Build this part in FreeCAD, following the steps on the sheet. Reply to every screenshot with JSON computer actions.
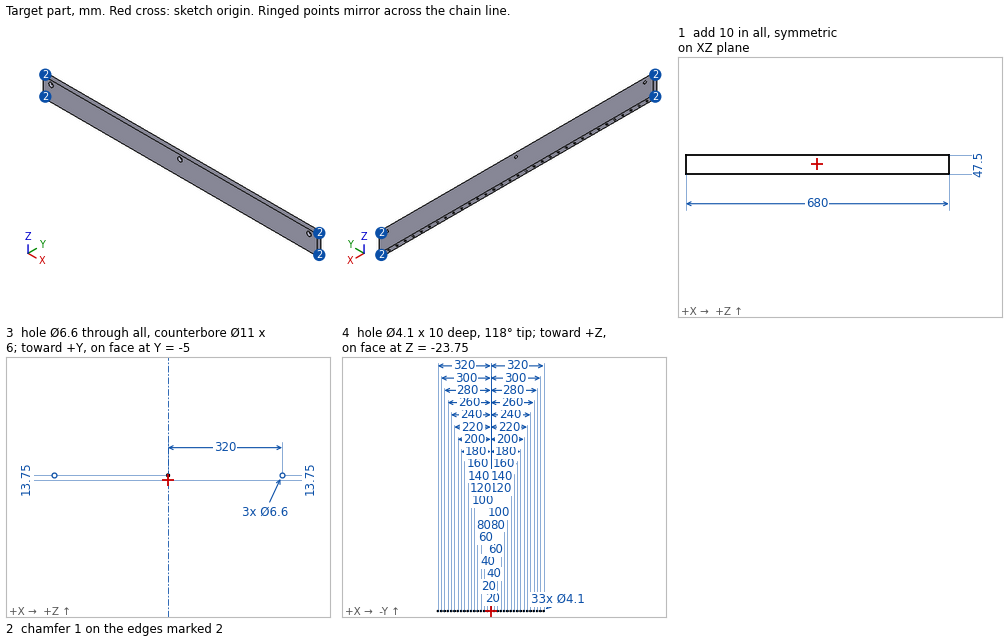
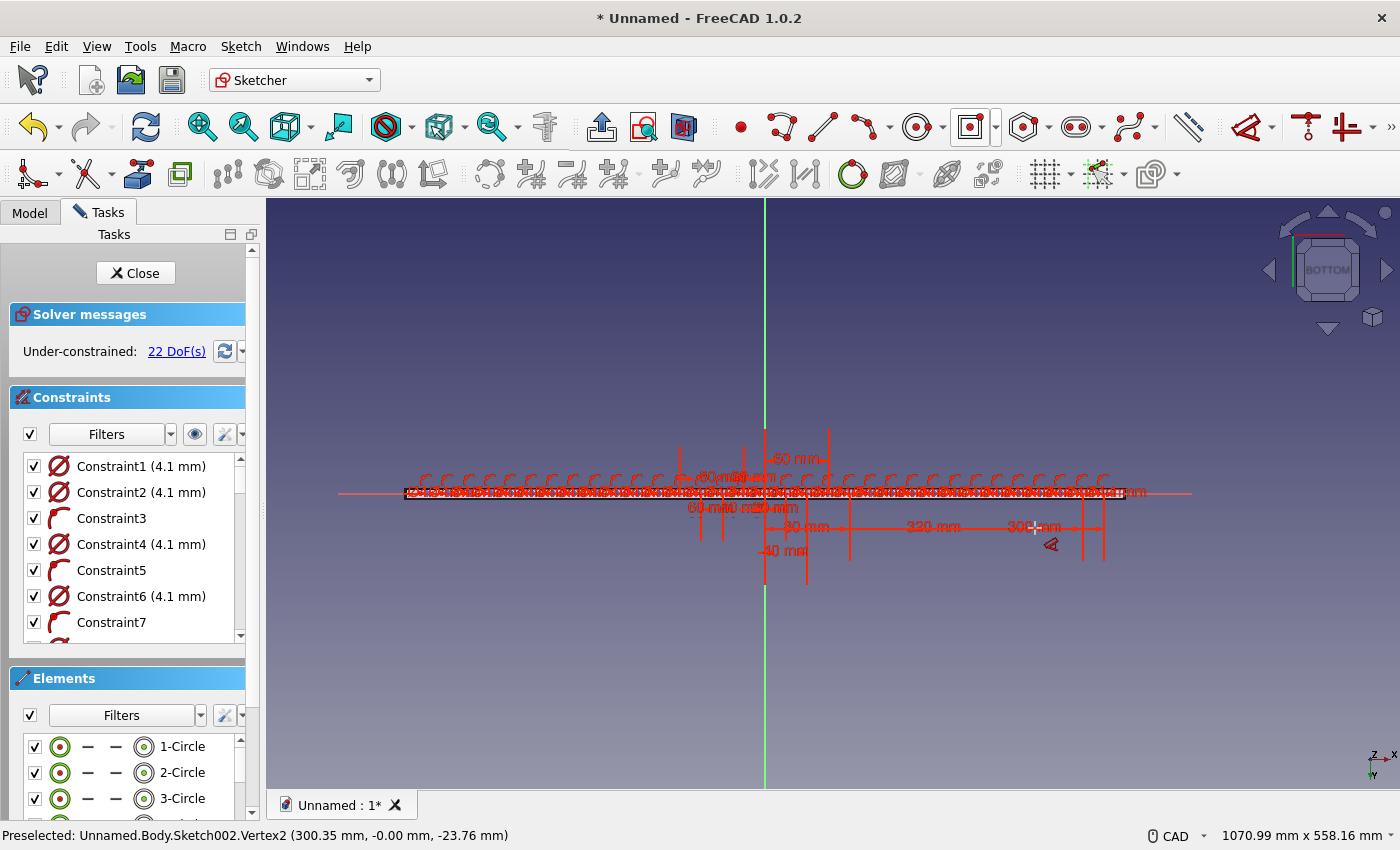
{"action": "left_click", "coordinate": [1061, 494]}
{"action": "left_click", "coordinate": [913, 460]}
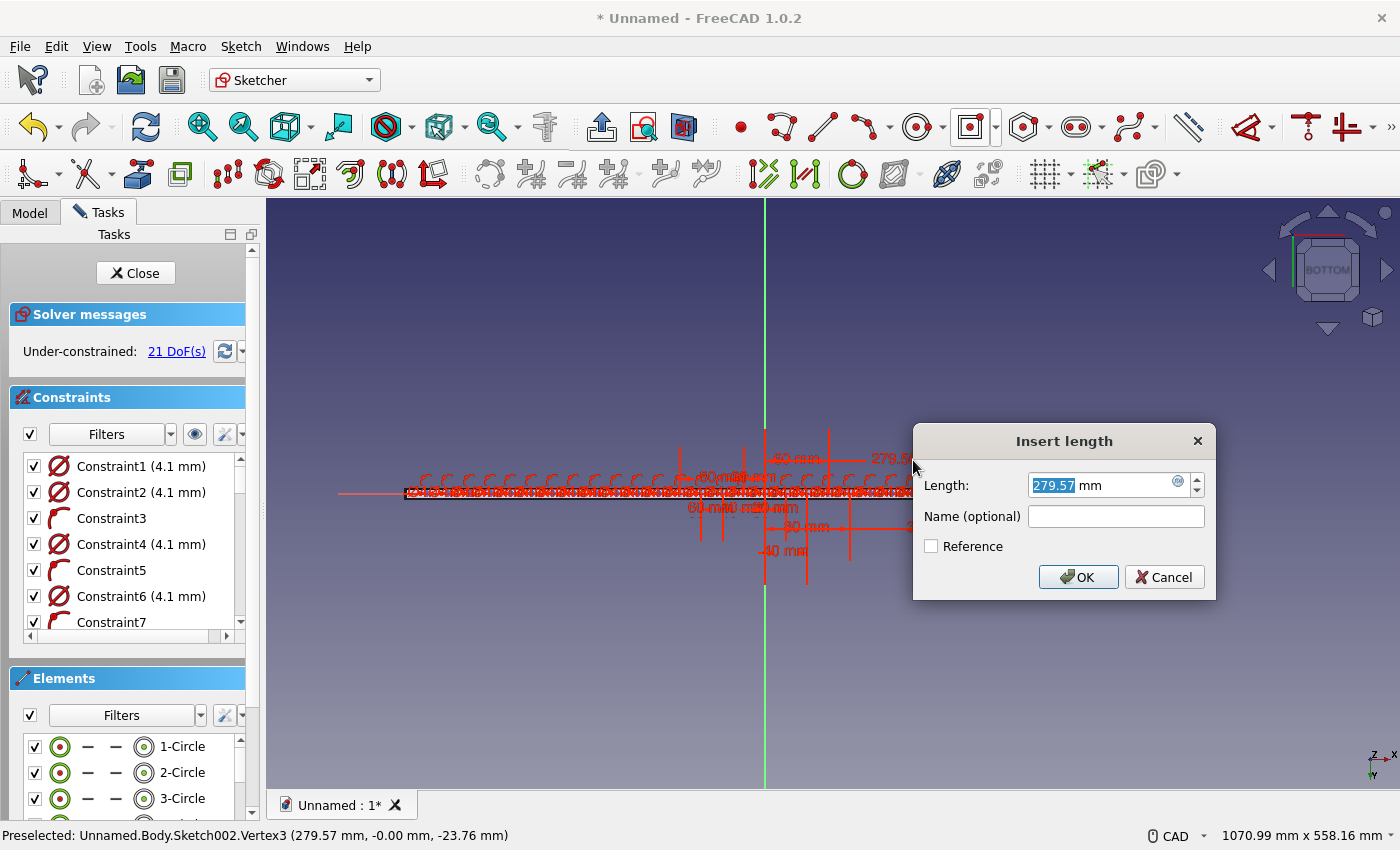
{"action": "type", "text": "280"}
{"action": "key", "text": "Return"}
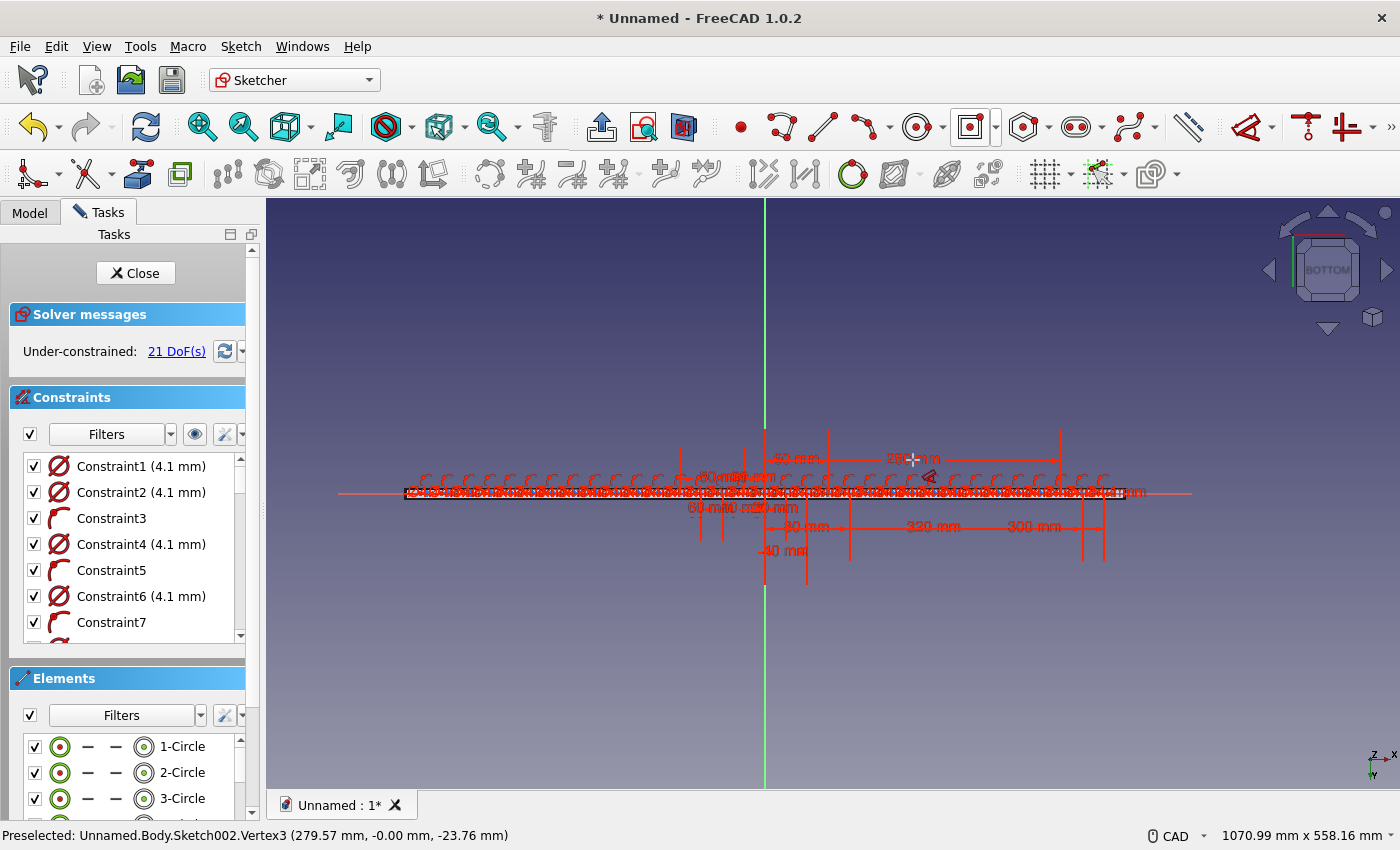
{"action": "left_click", "coordinate": [1040, 494]}
{"action": "left_click", "coordinate": [999, 460]}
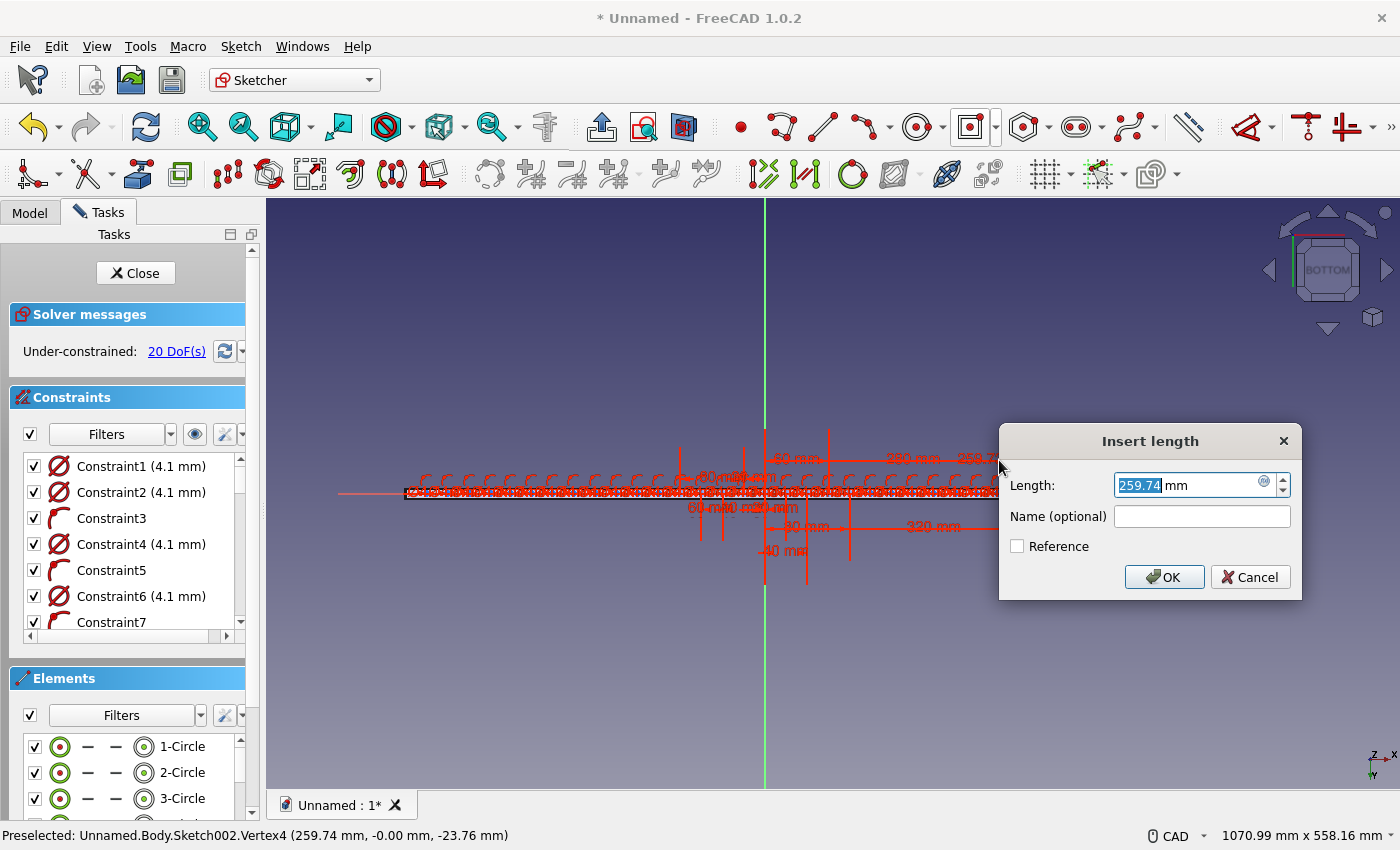
{"action": "type", "text": "260"}
{"action": "key", "text": "Return"}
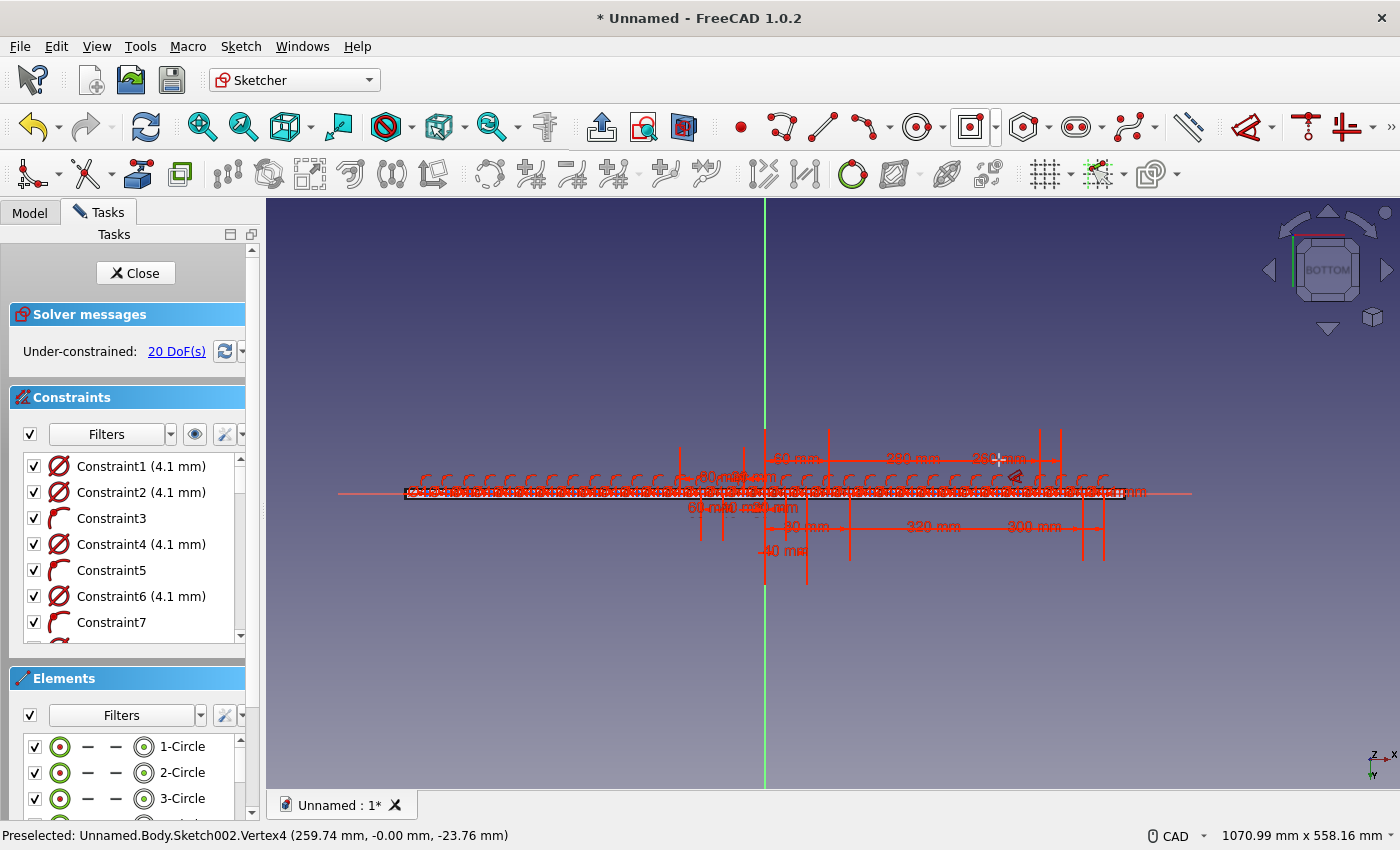
{"action": "left_click", "coordinate": [1019, 494]}
{"action": "left_click", "coordinate": [892, 552]}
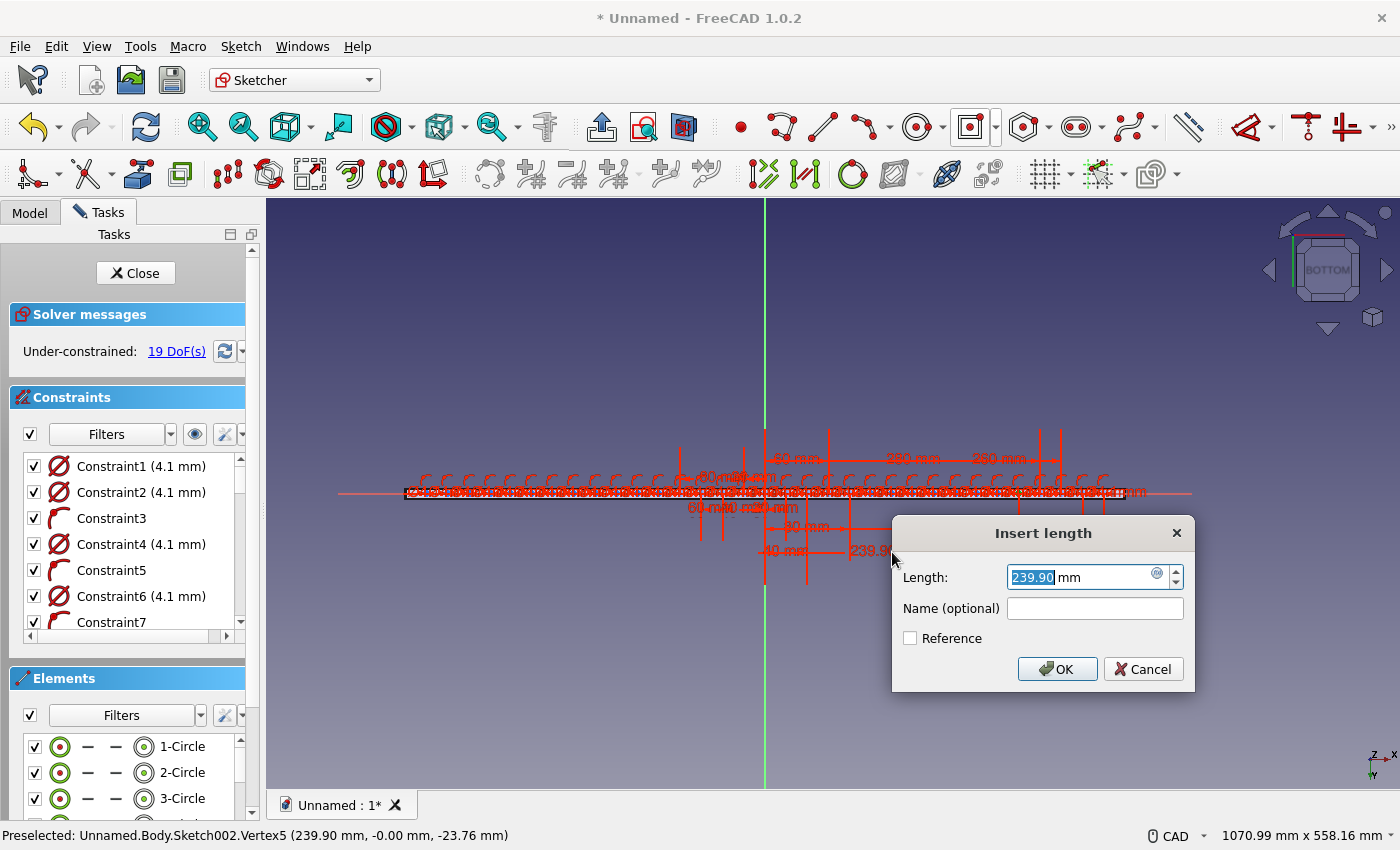
{"action": "type", "text": "240"}
{"action": "key", "text": "Return"}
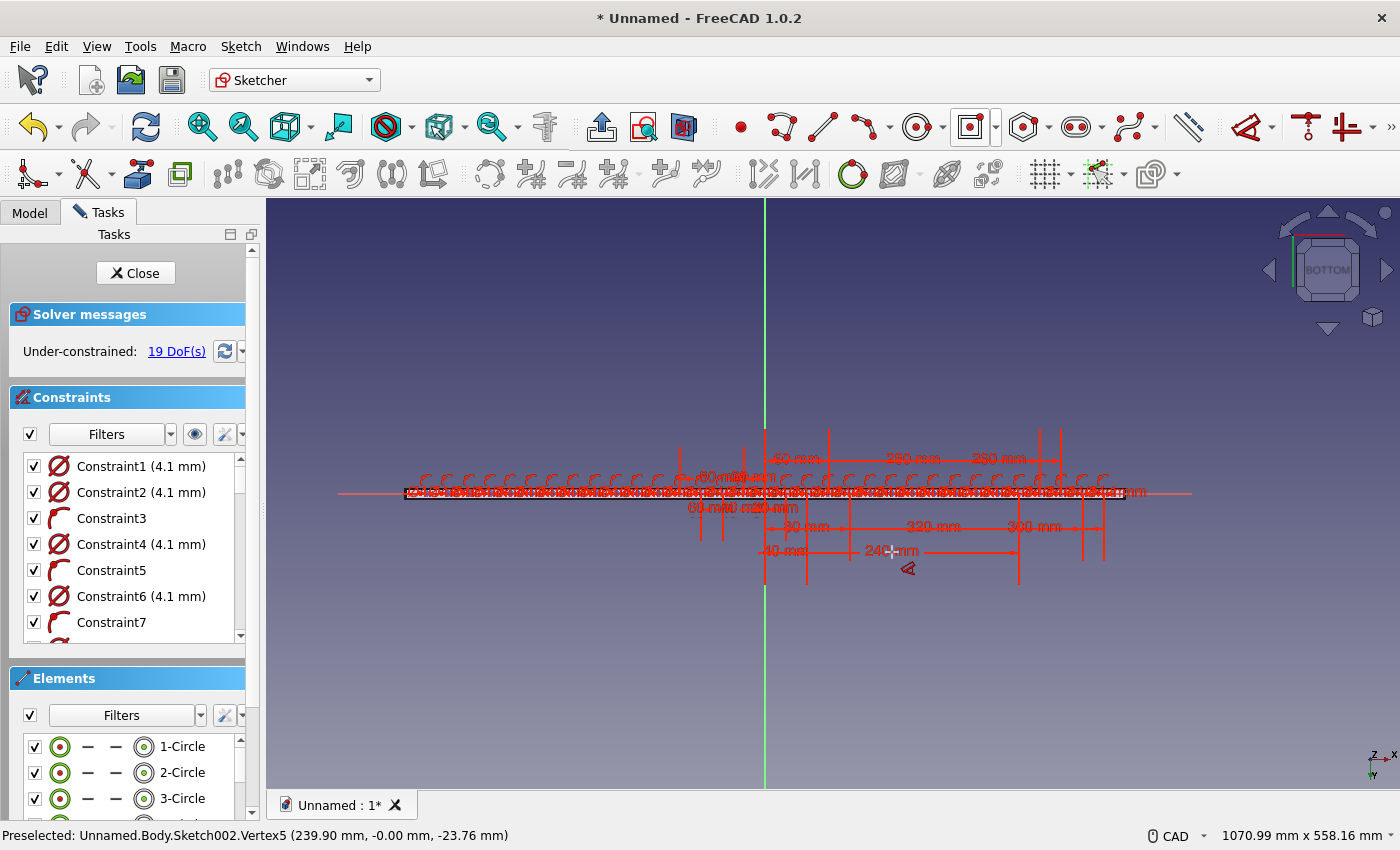
{"action": "left_click", "coordinate": [998, 494]}
{"action": "left_click", "coordinate": [963, 552]}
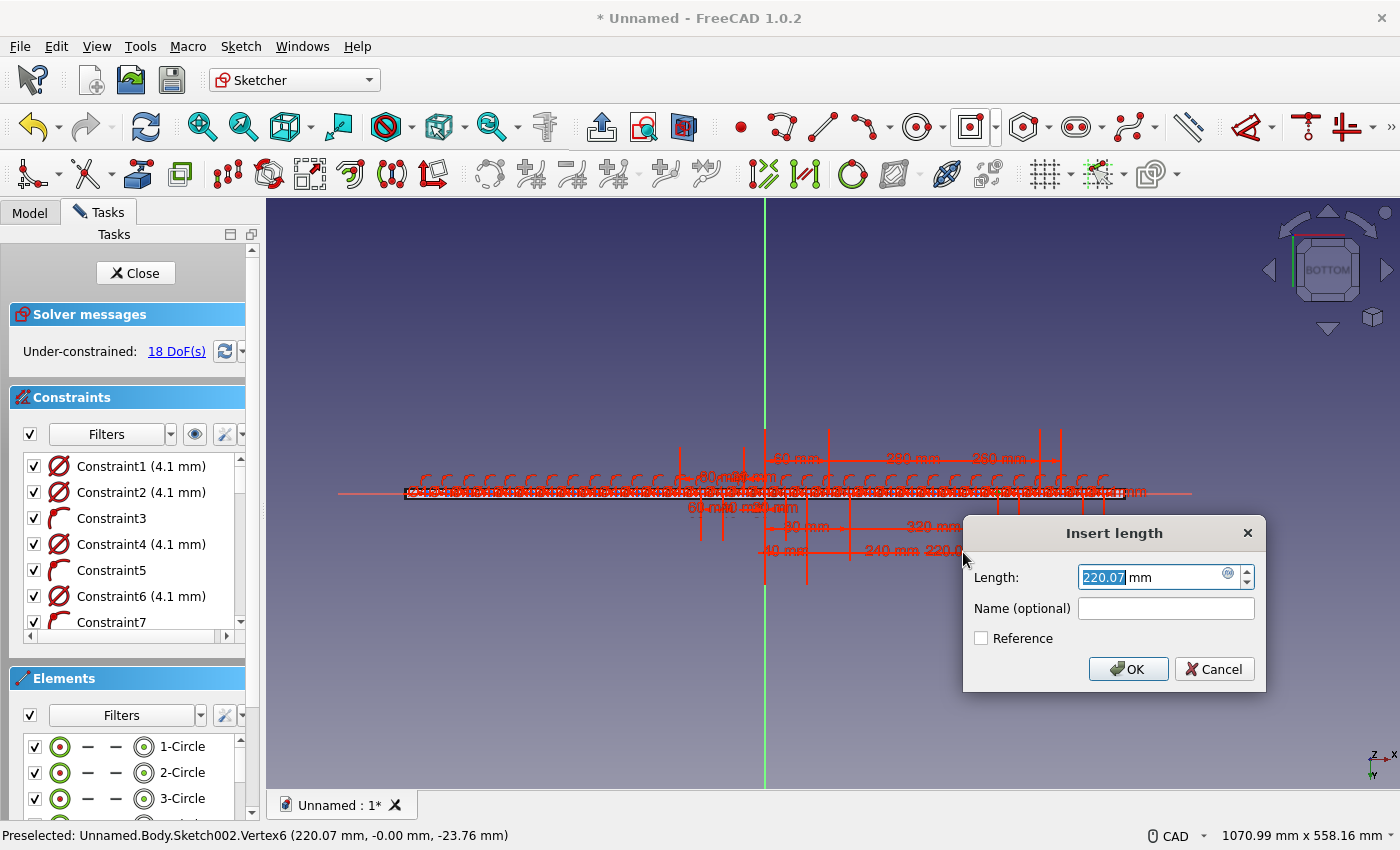
{"action": "type", "text": "220"}
{"action": "key", "text": "Return"}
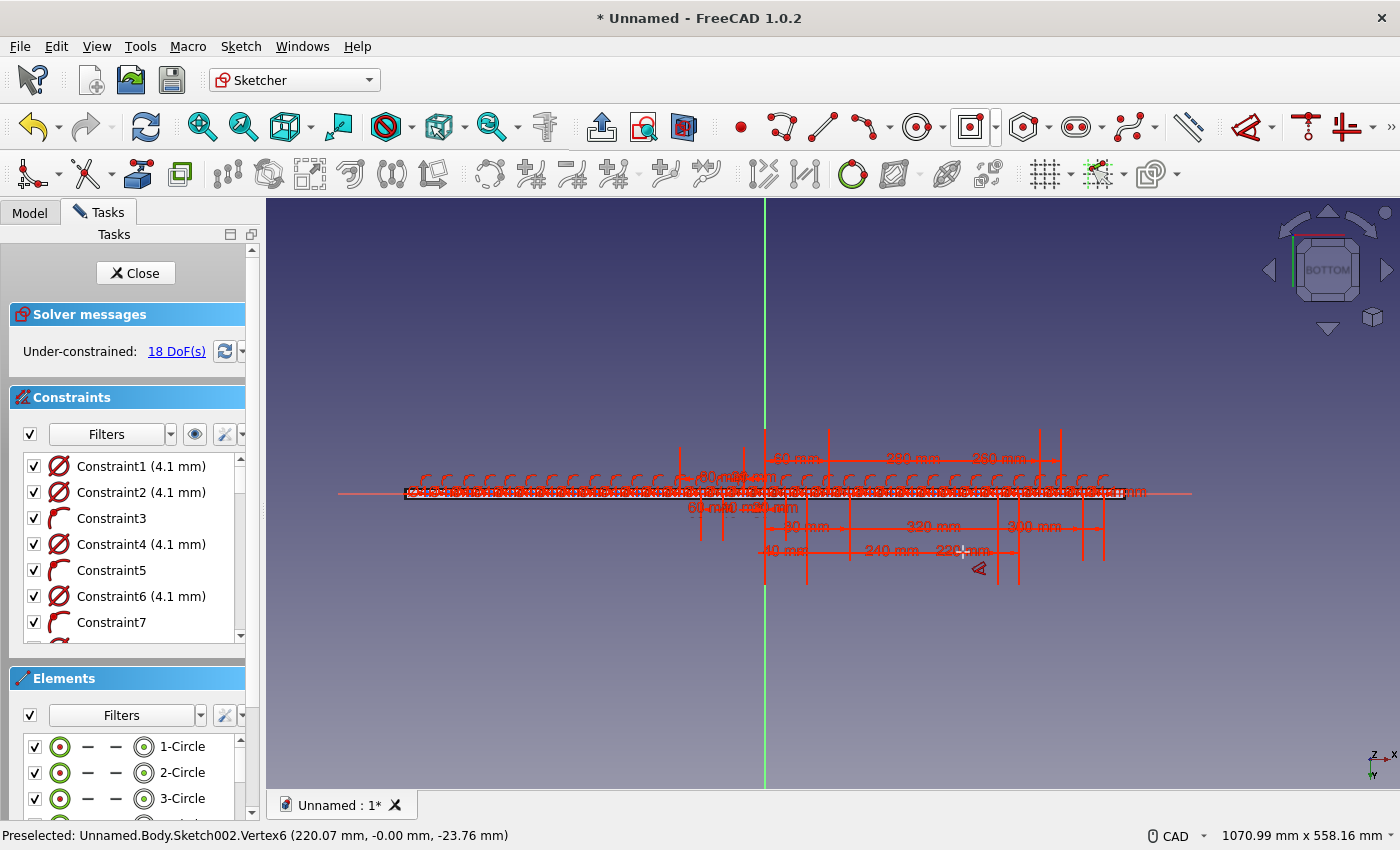
{"action": "left_click", "coordinate": [977, 494]}
{"action": "left_click", "coordinate": [871, 436]}